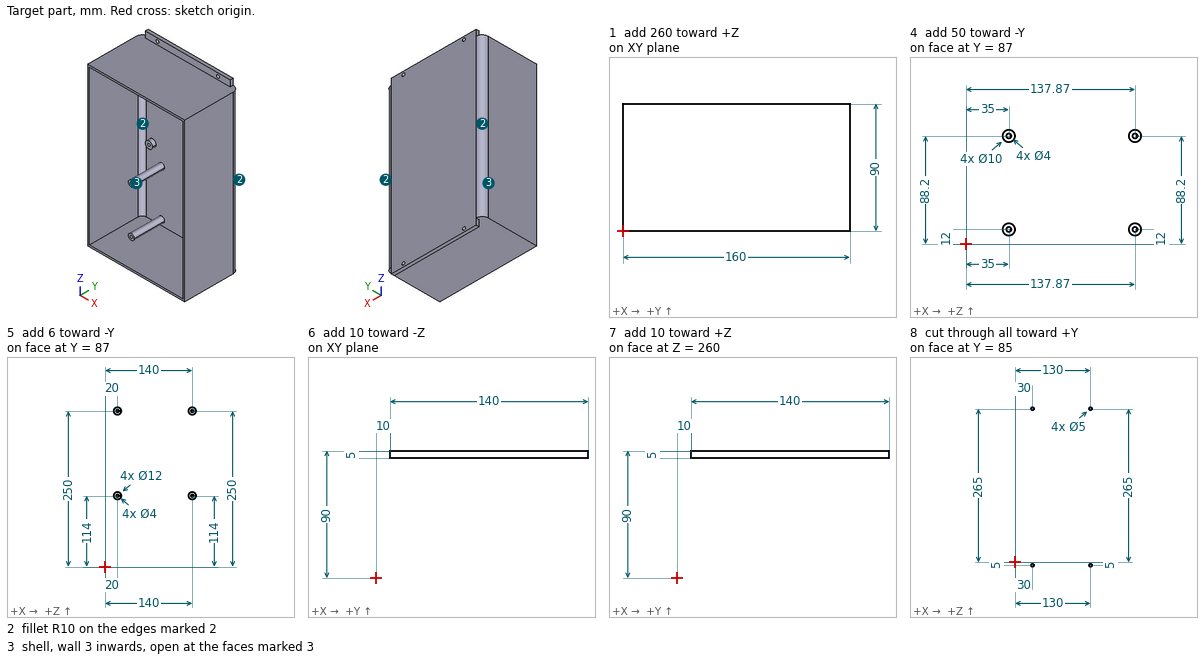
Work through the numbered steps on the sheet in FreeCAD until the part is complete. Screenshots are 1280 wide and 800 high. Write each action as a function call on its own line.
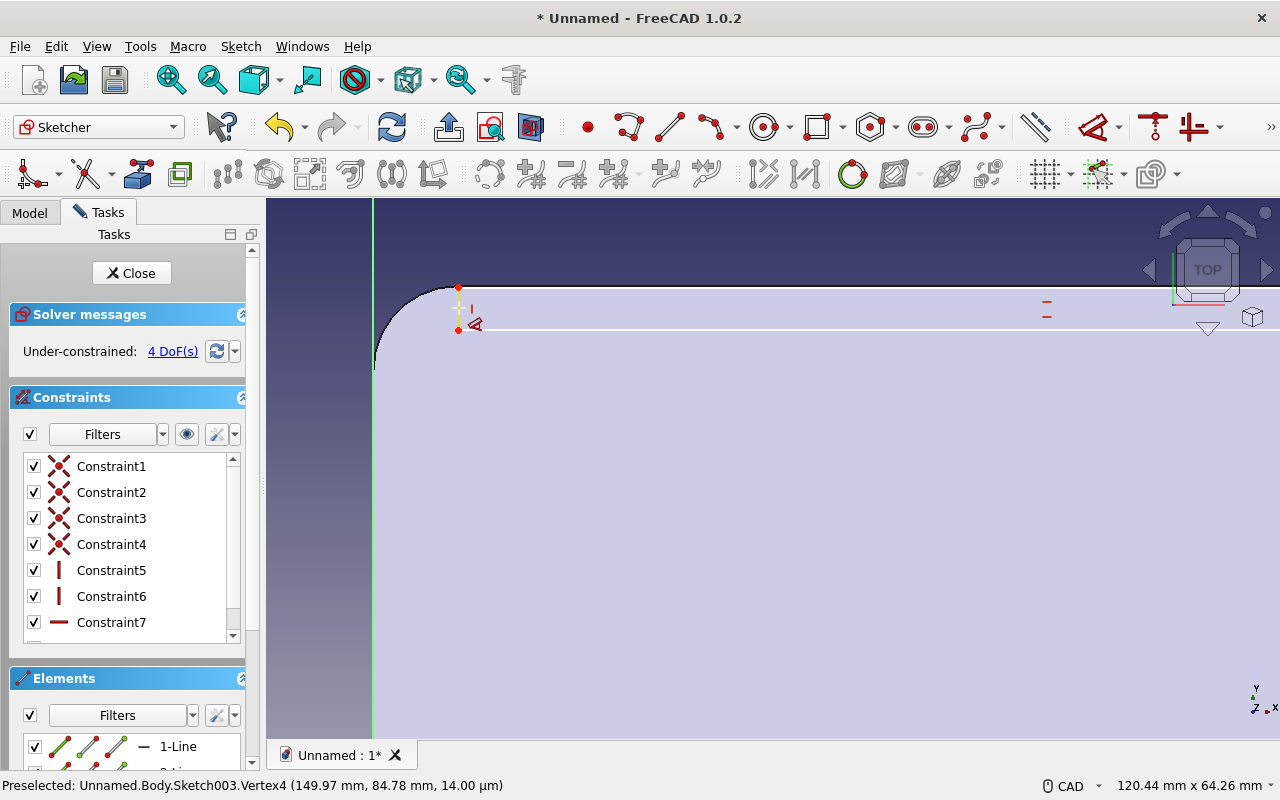
click(459, 309)
click(425, 309)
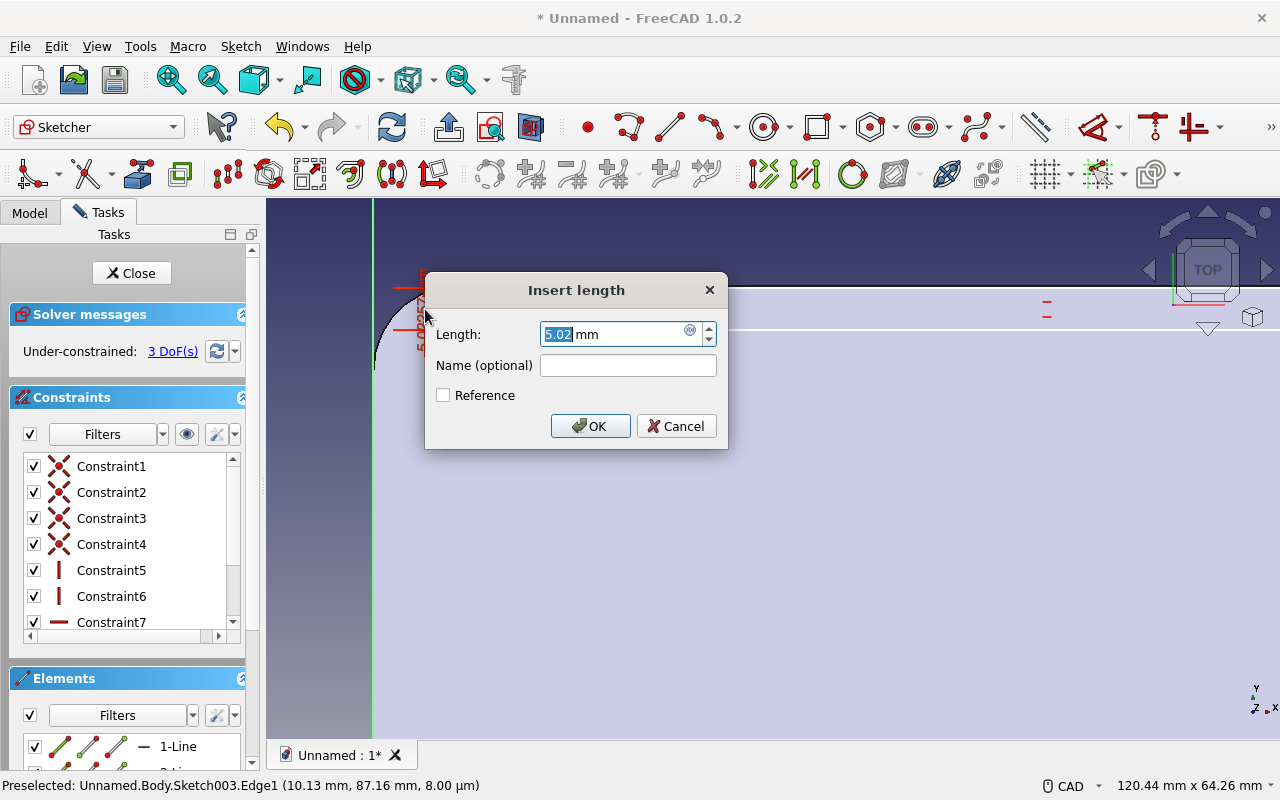
text(5)
key(Return)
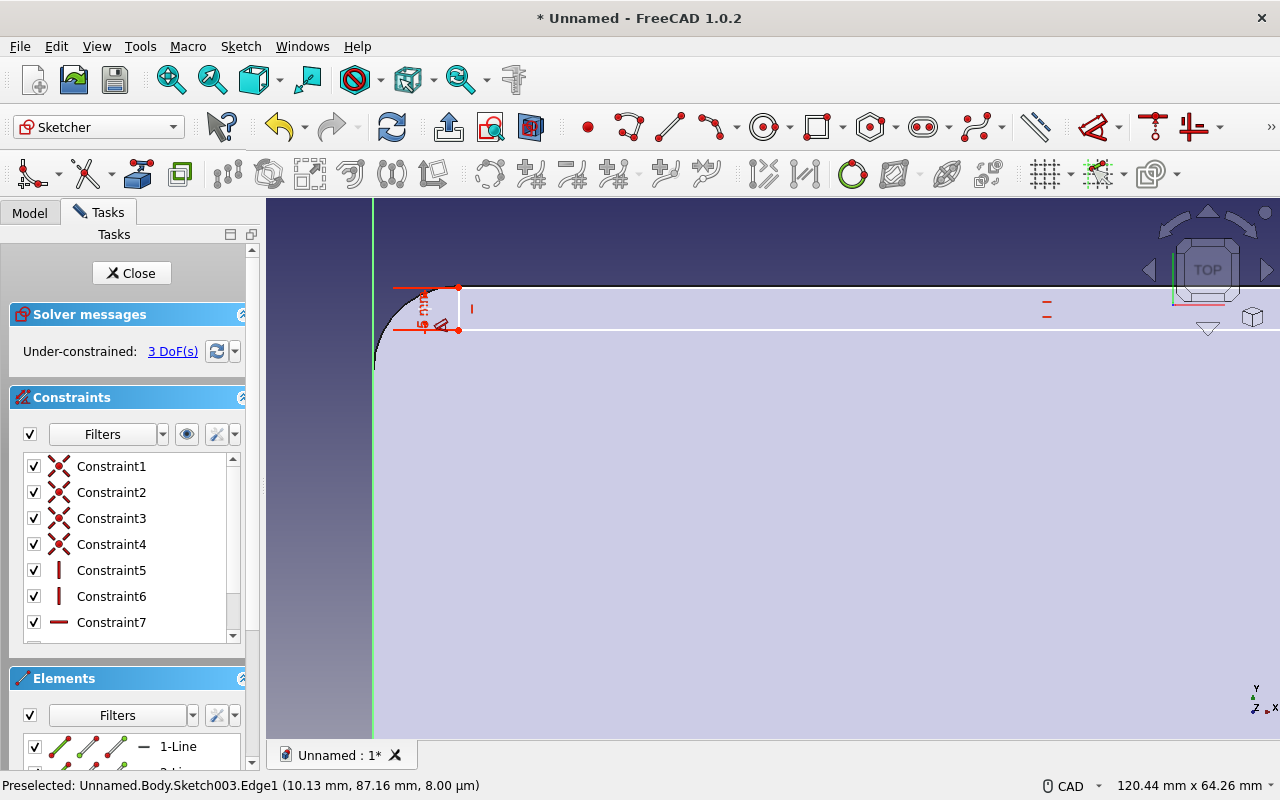
click(812, 330)
click(787, 364)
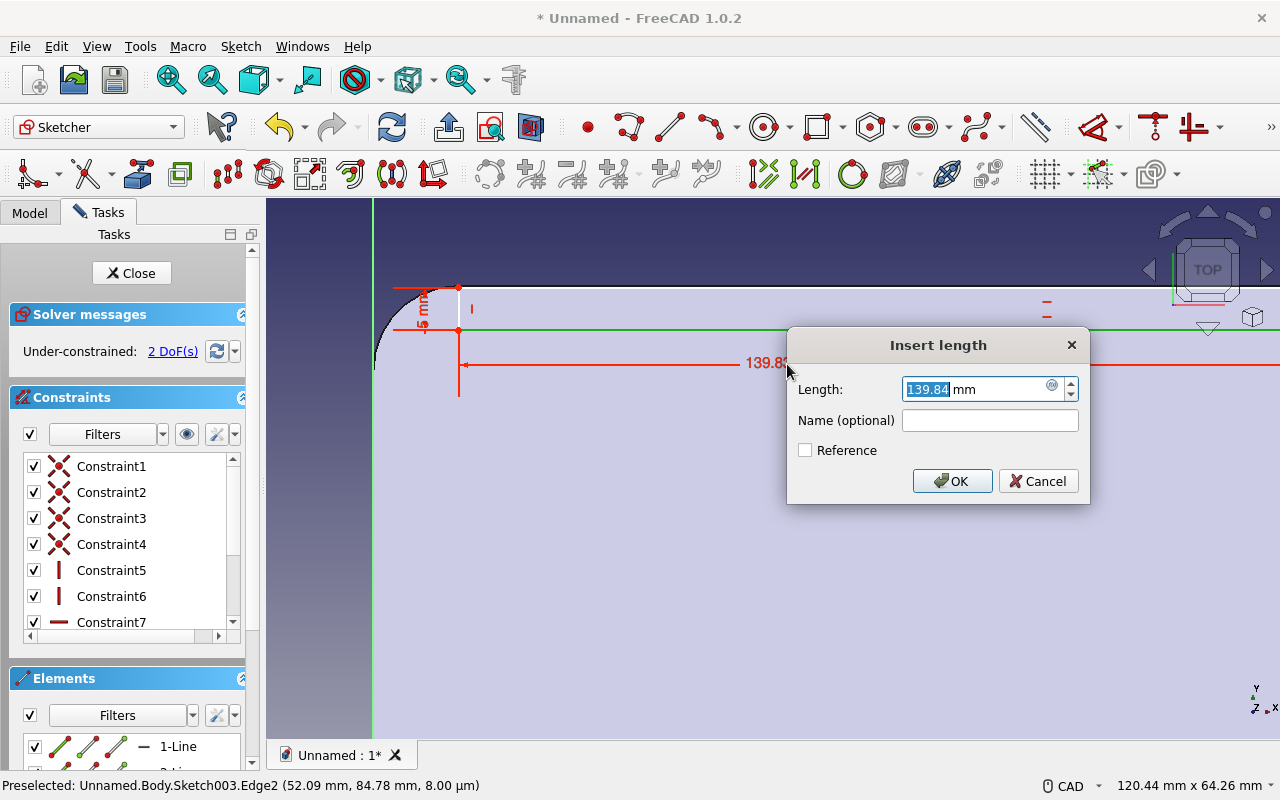
text(140)
key(Return)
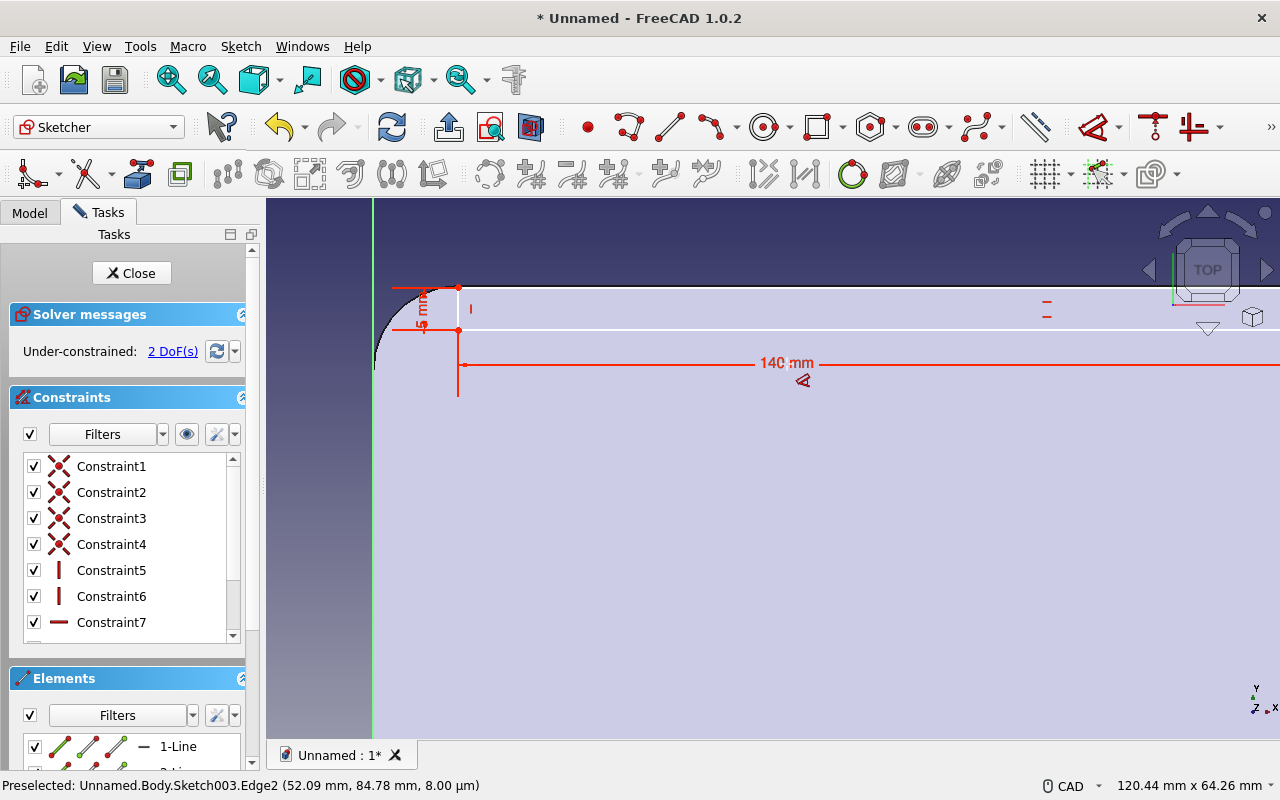
click(458, 288)
click(416, 254)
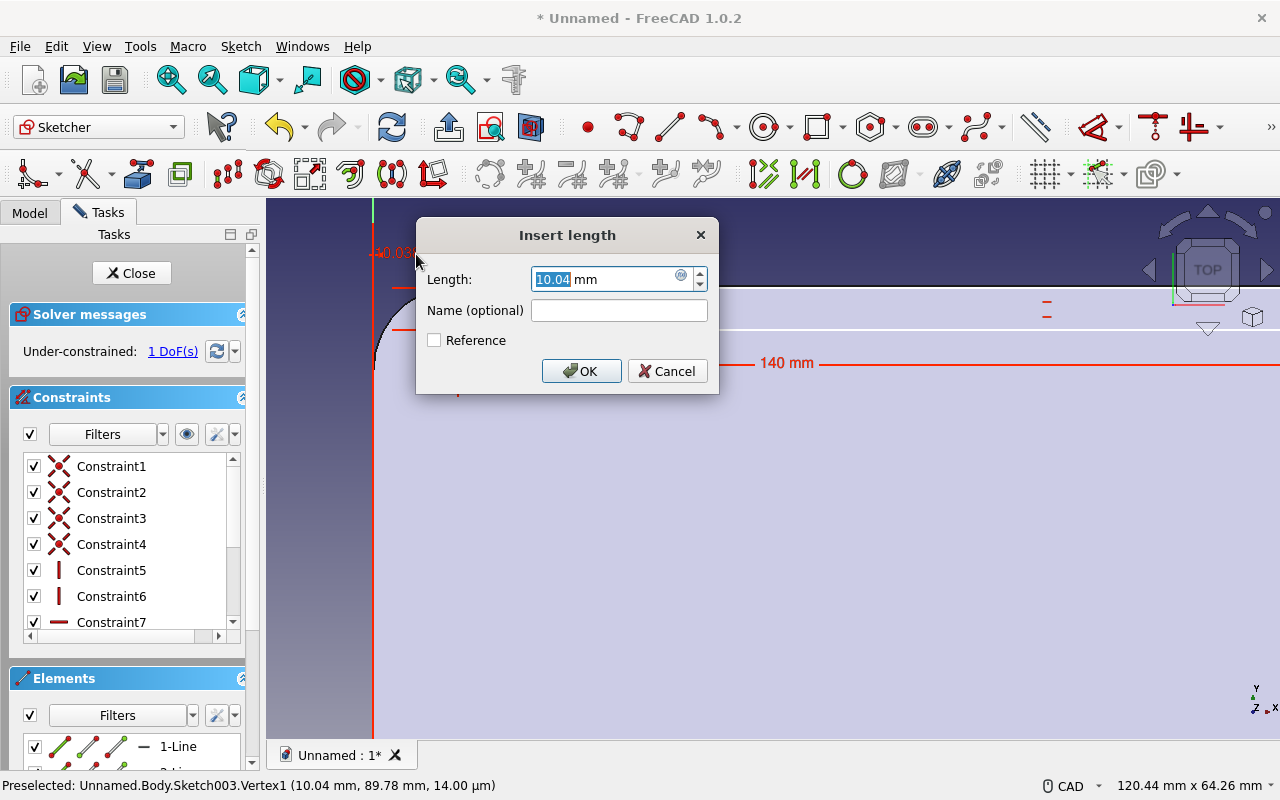
text(10)
key(Return)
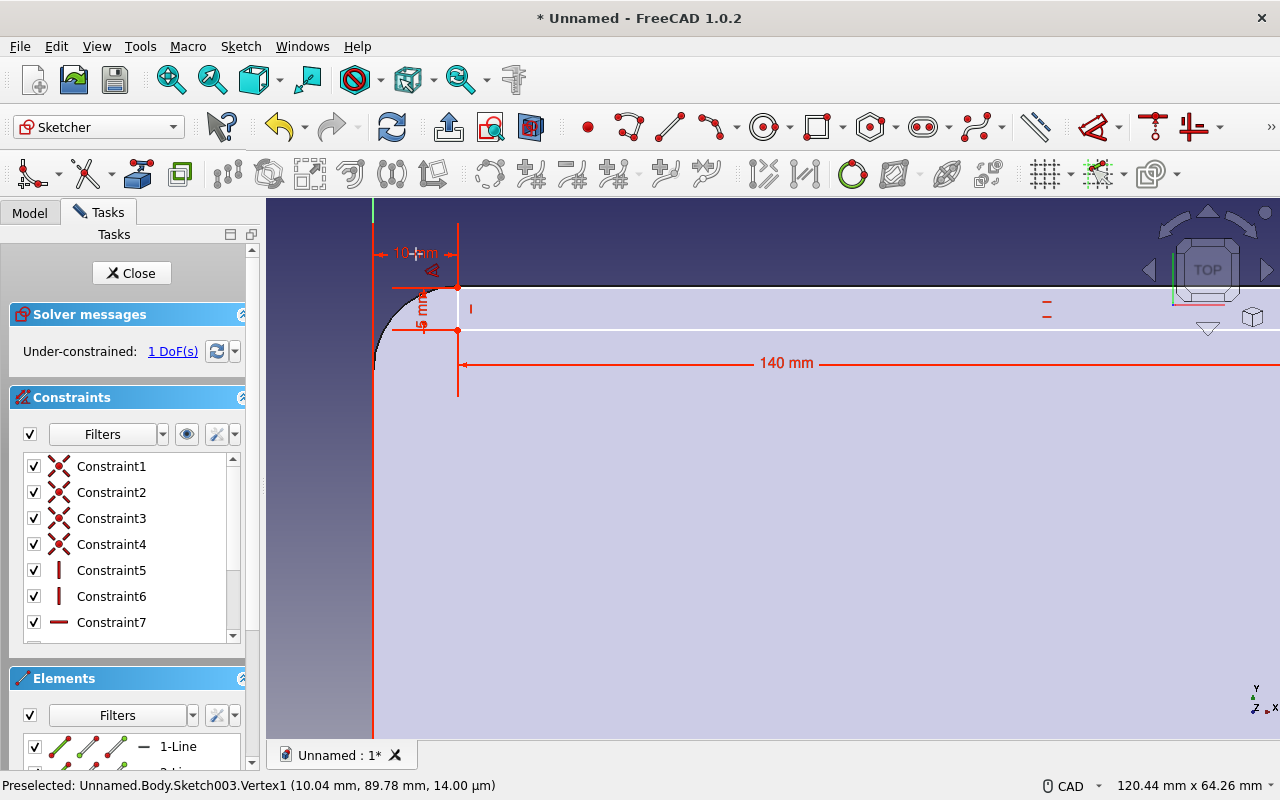
click(458, 288)
click(339, 499)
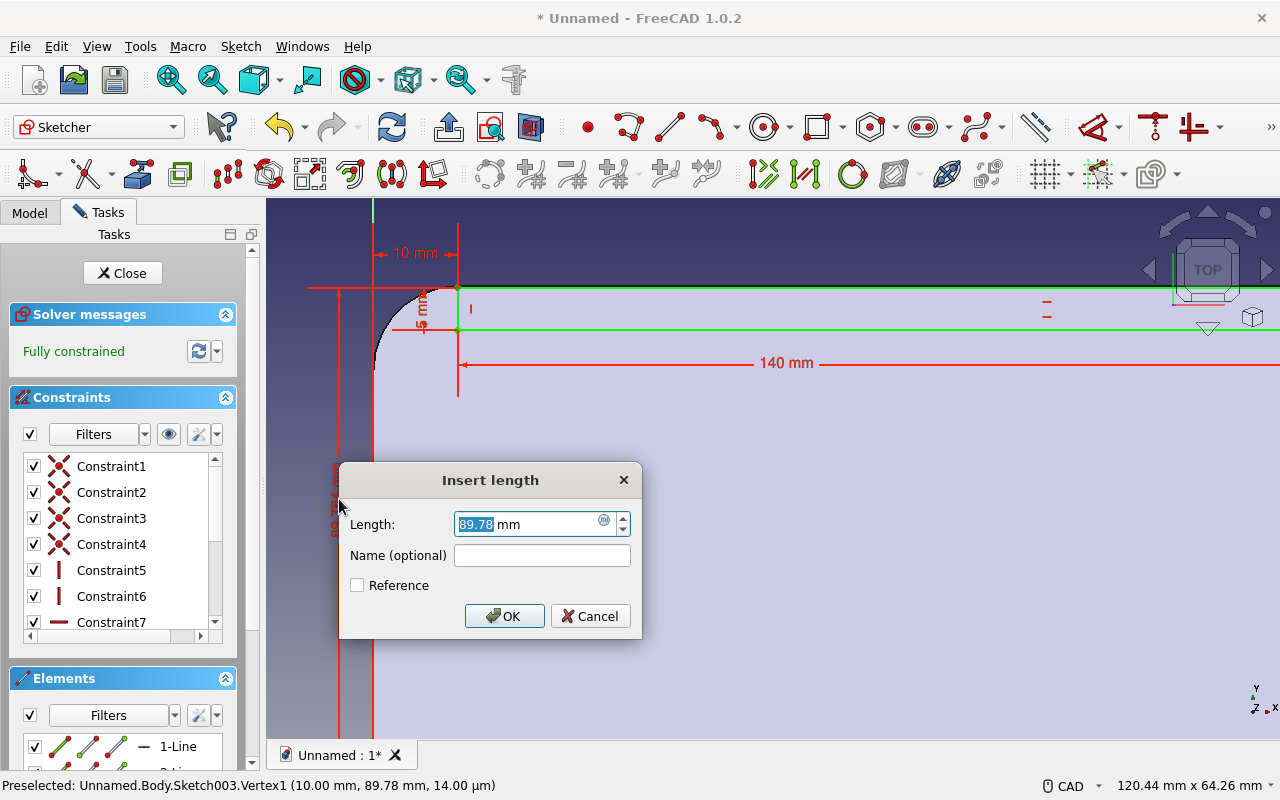
text(90)
key(Return)
key(Escape)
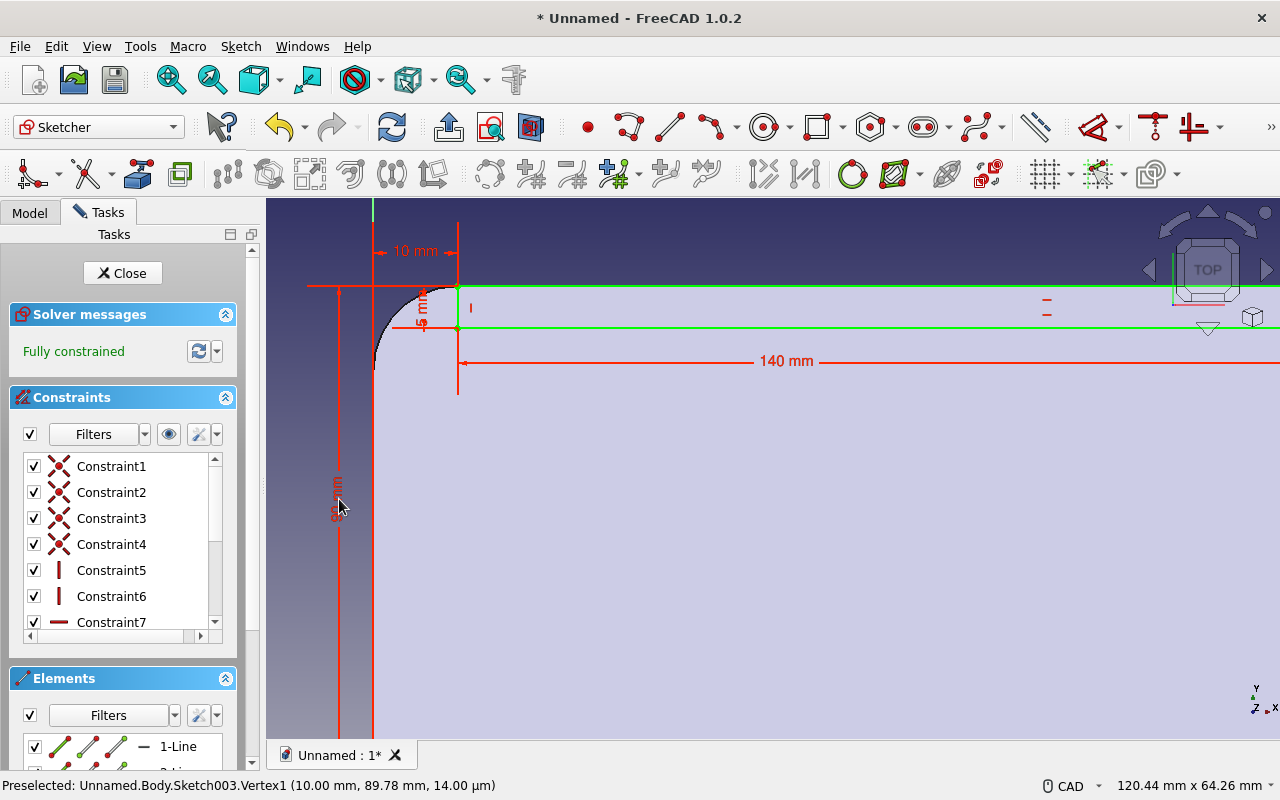
click(123, 273)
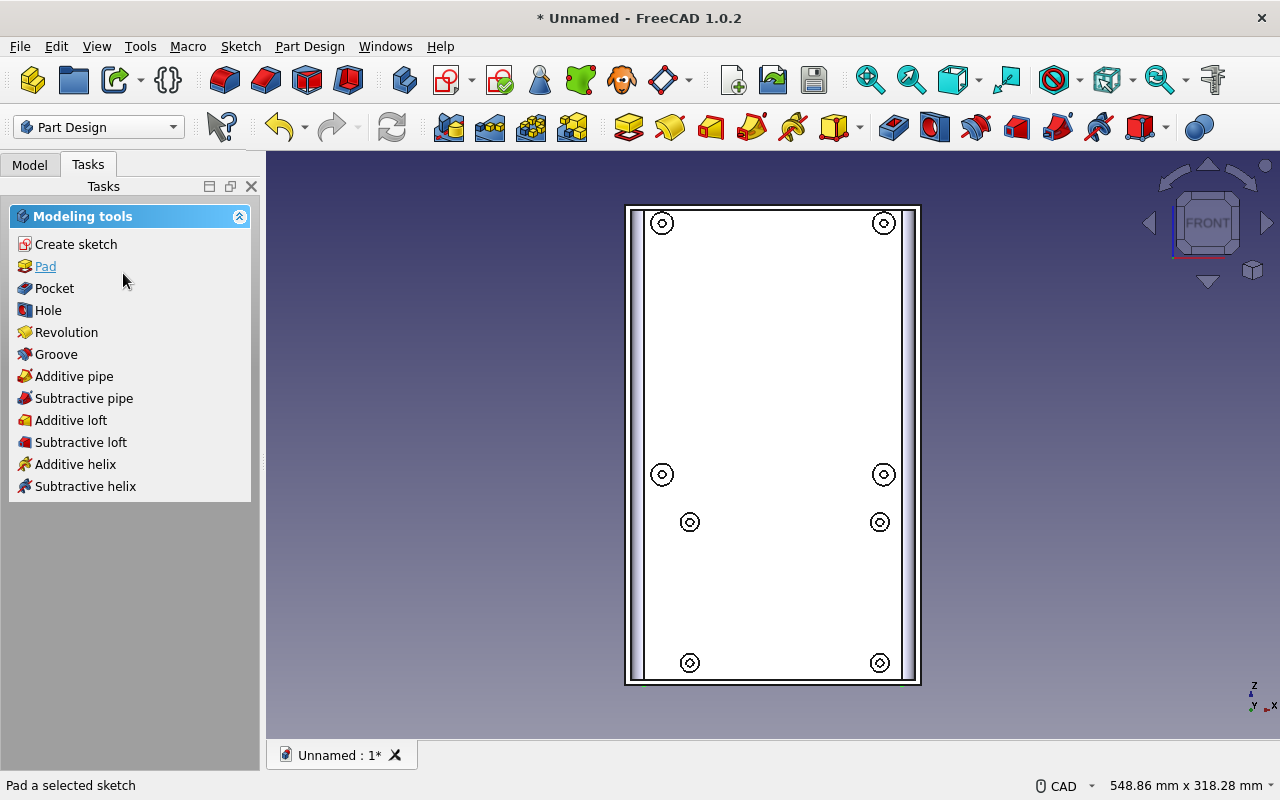
click(629, 128)